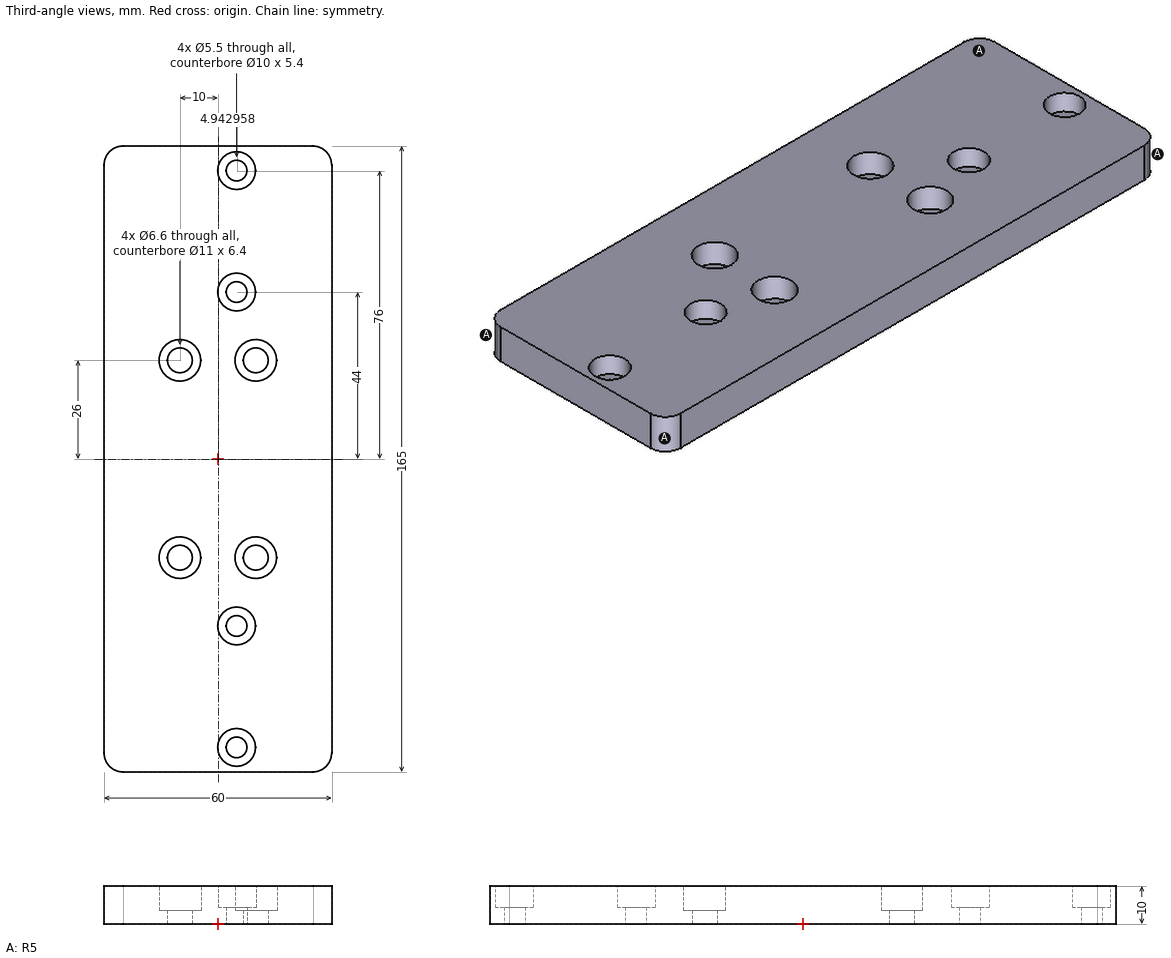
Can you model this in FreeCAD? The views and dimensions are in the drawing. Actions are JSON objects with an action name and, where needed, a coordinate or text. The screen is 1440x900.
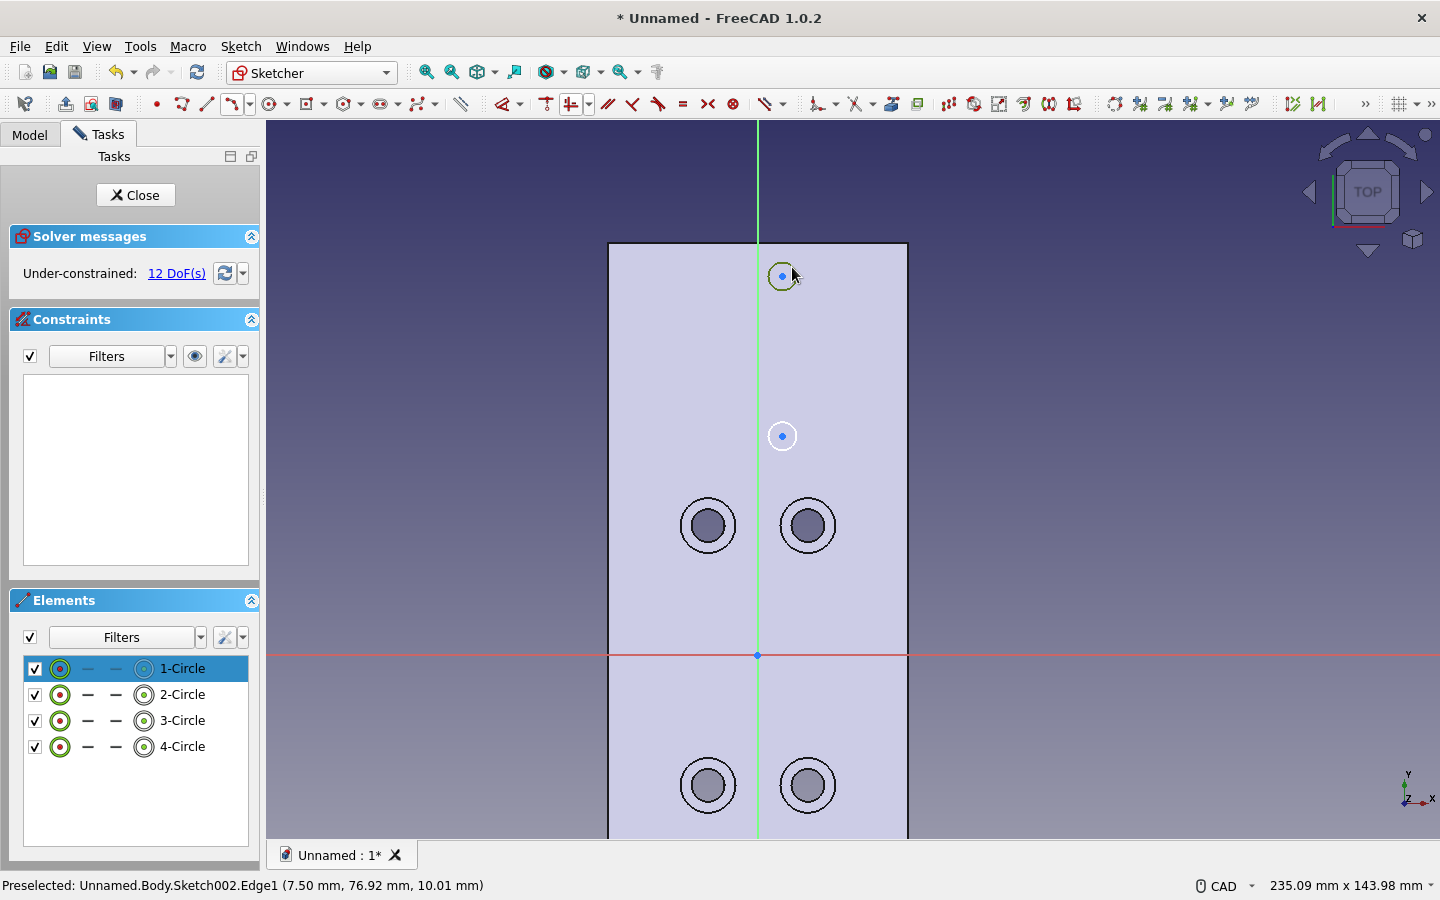
{"action": "left_click", "coordinate": [792, 426]}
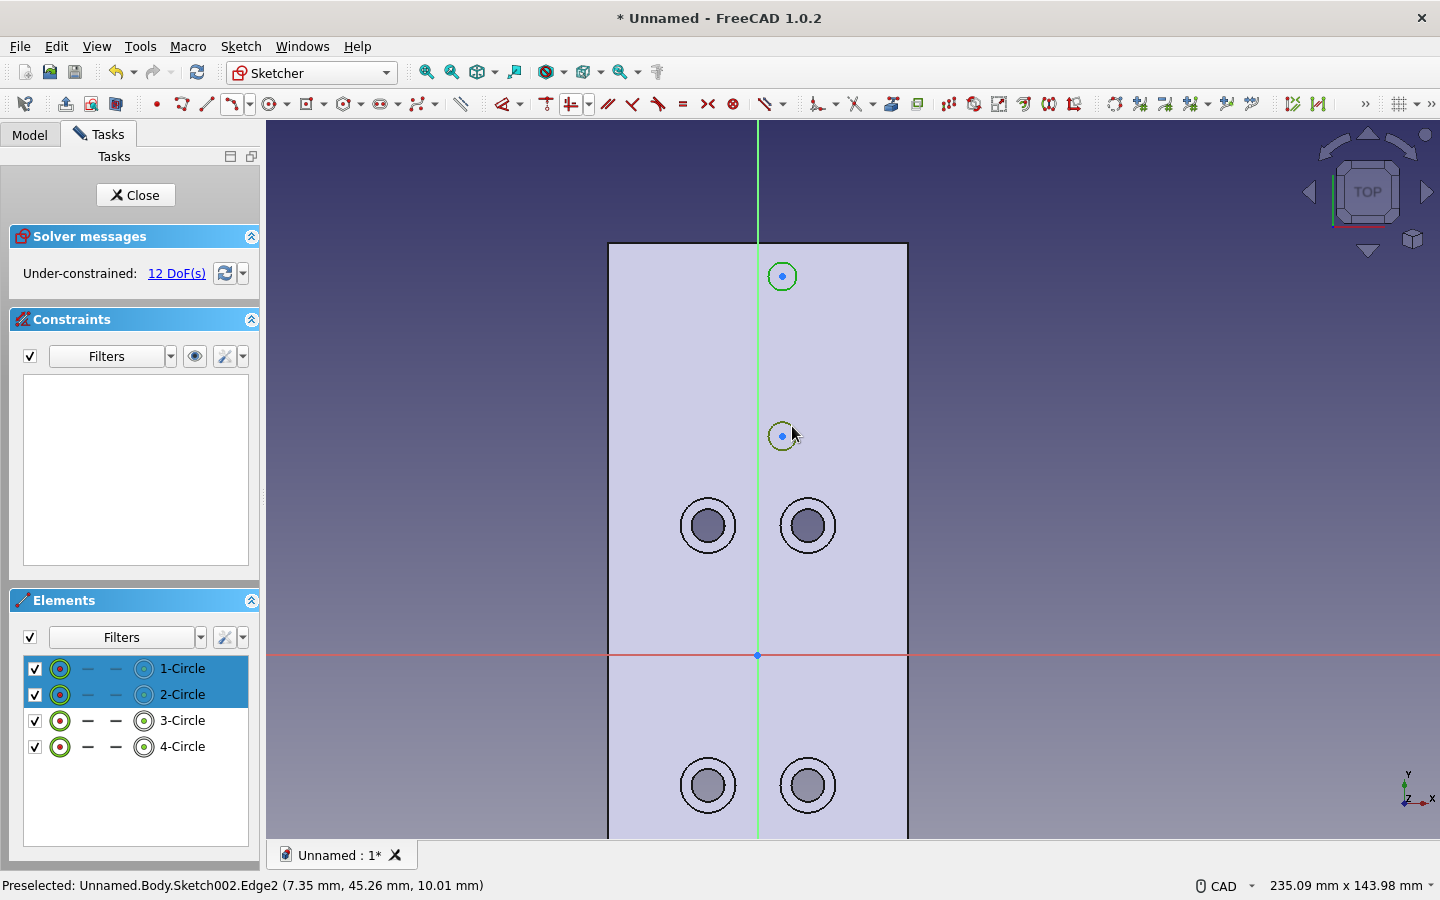
{"action": "scroll", "coordinate": [793, 265], "scroll_direction": "down", "scroll_amount": 3}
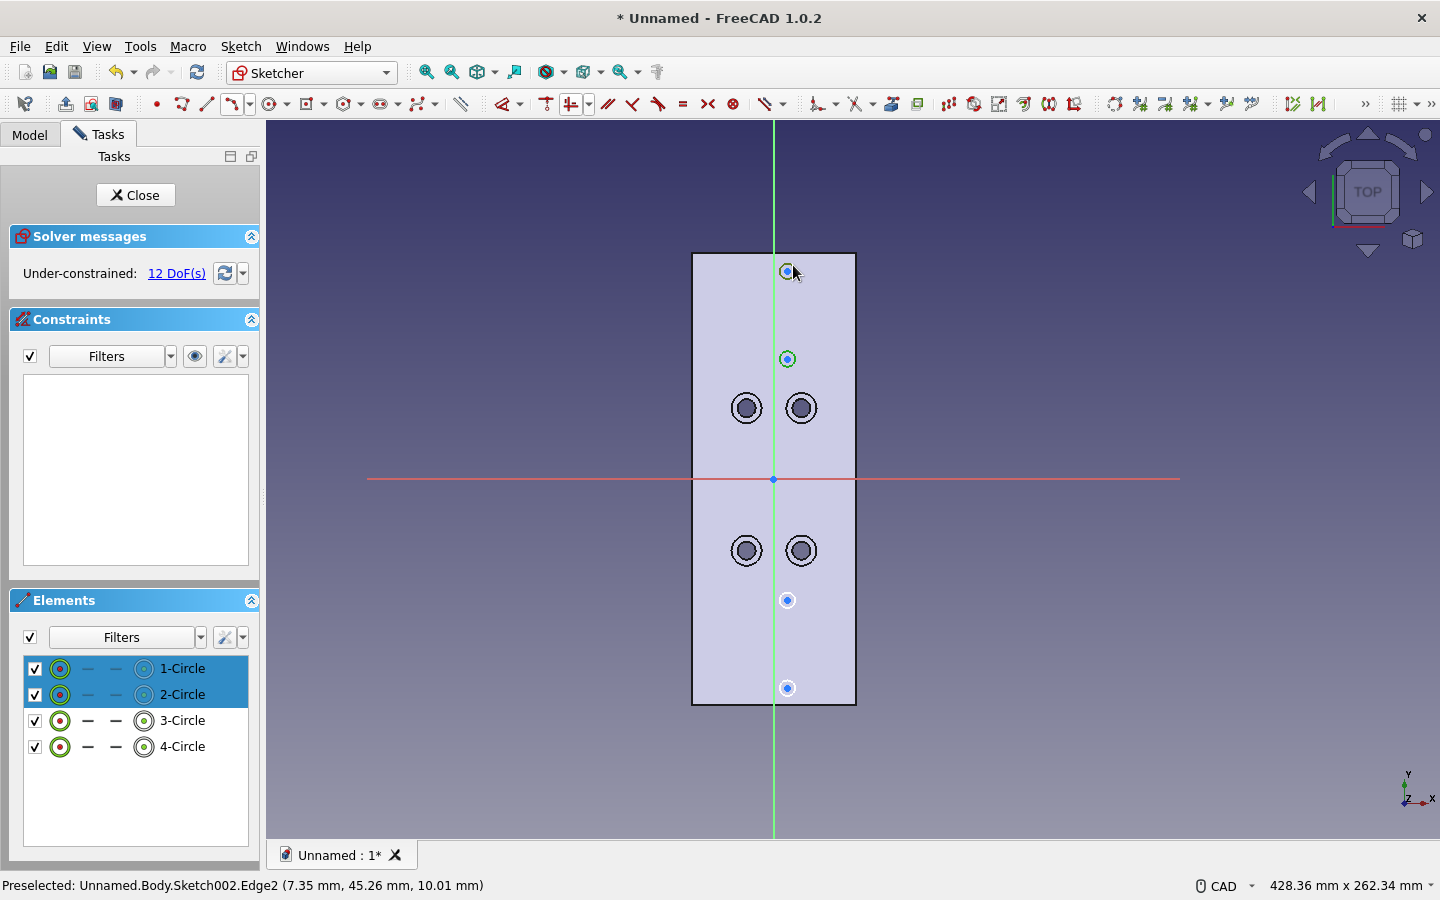
{"action": "scroll", "coordinate": [793, 595], "scroll_direction": "up", "scroll_amount": 3}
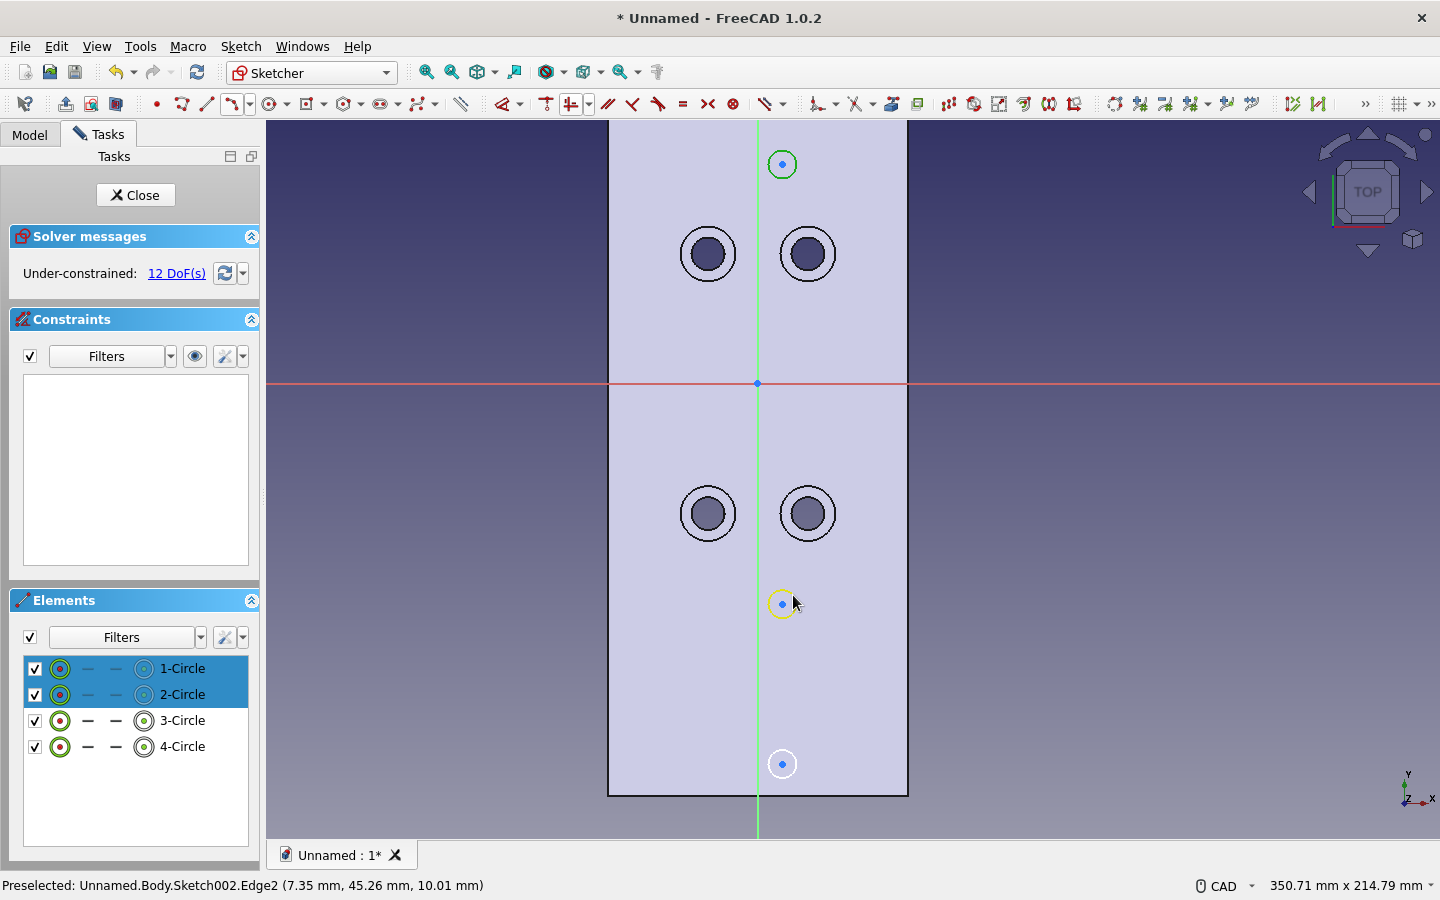
{"action": "left_click", "coordinate": [792, 594]}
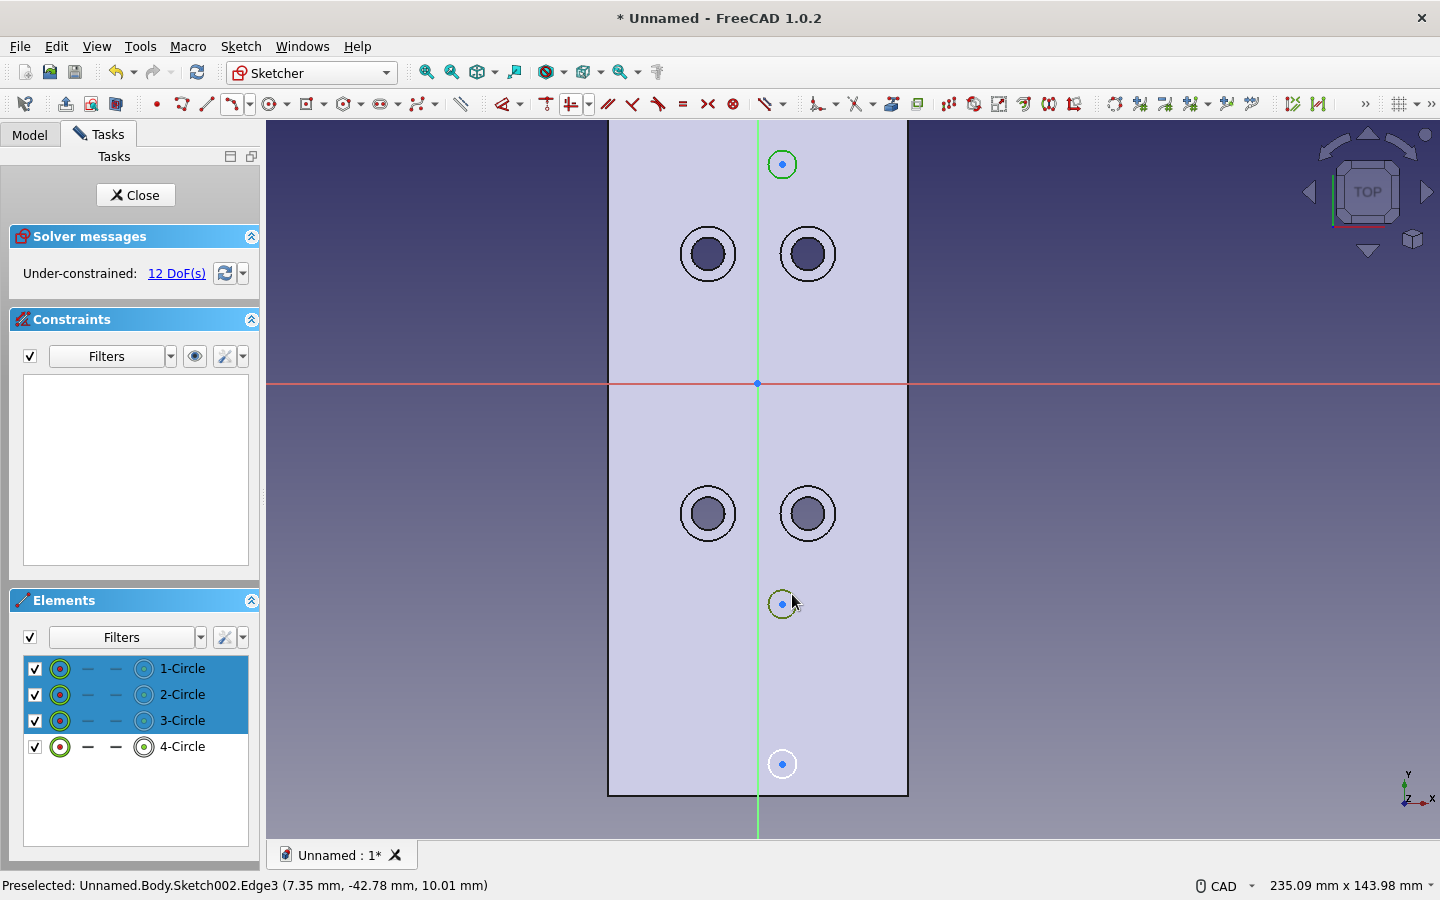
{"action": "left_click", "coordinate": [792, 754]}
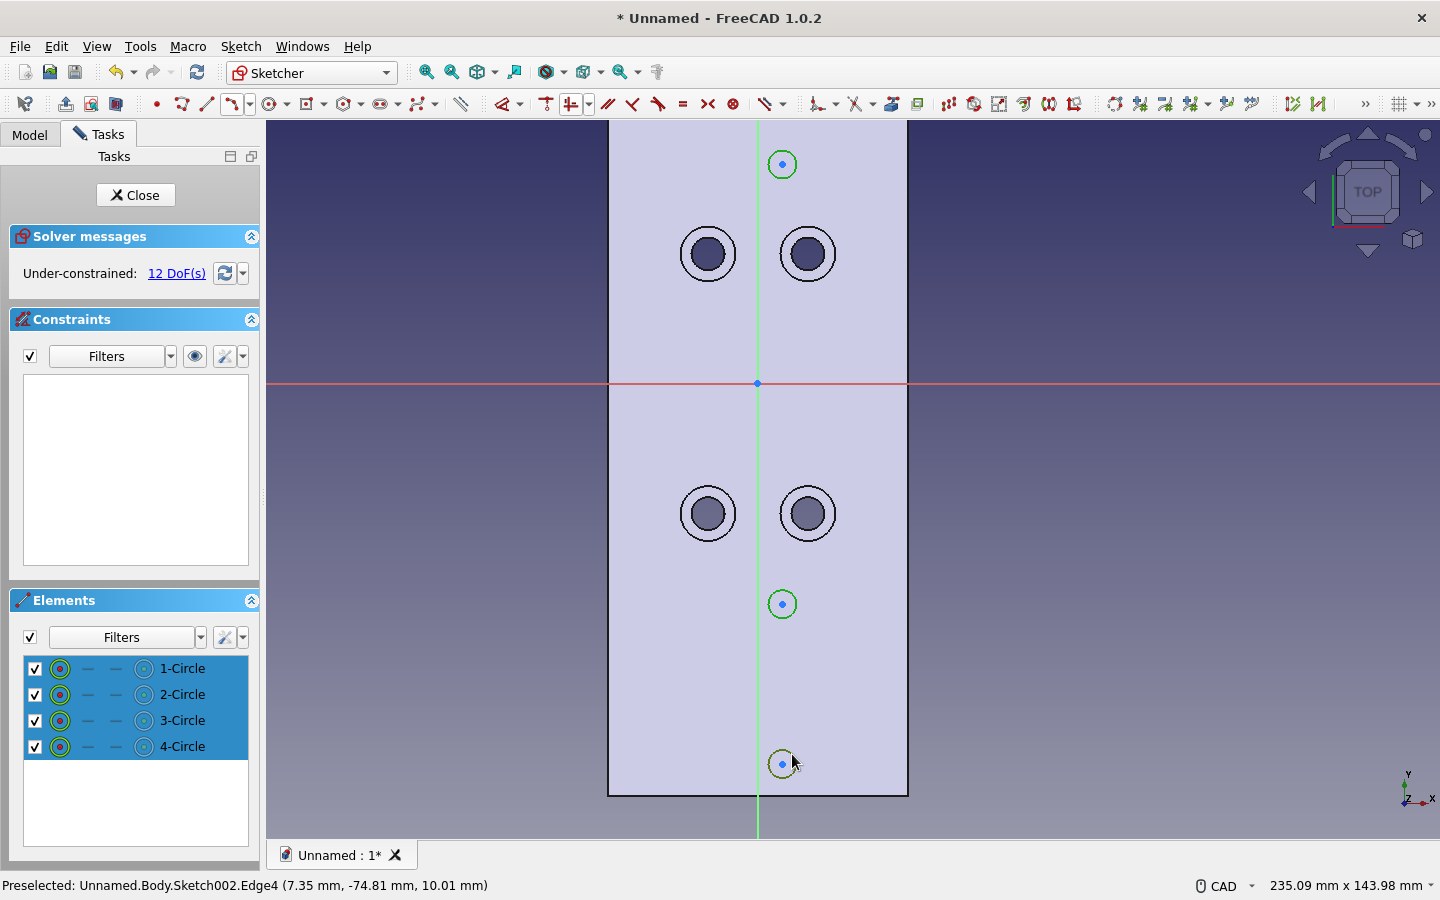
{"action": "left_click", "coordinate": [683, 104]}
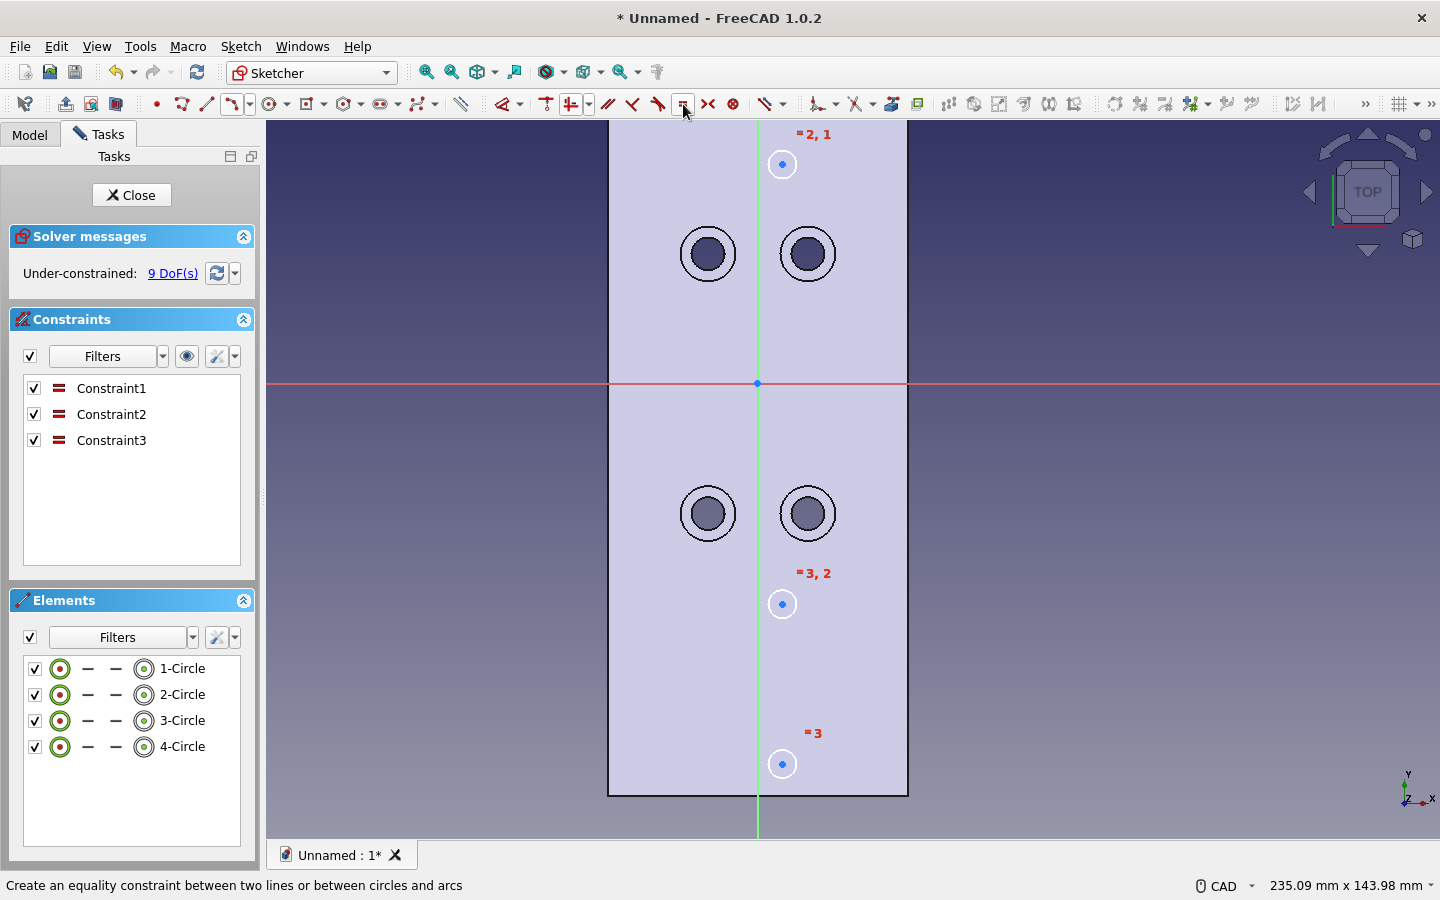
{"action": "left_click", "coordinate": [782, 165]}